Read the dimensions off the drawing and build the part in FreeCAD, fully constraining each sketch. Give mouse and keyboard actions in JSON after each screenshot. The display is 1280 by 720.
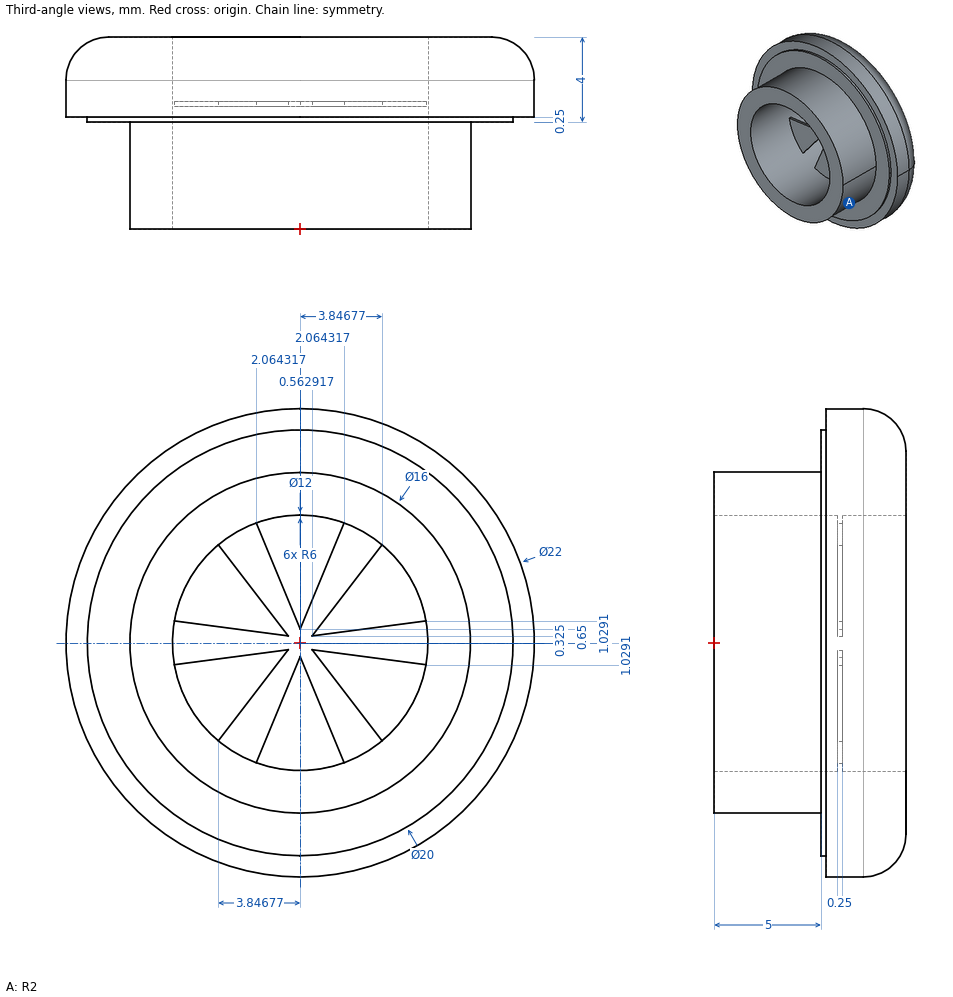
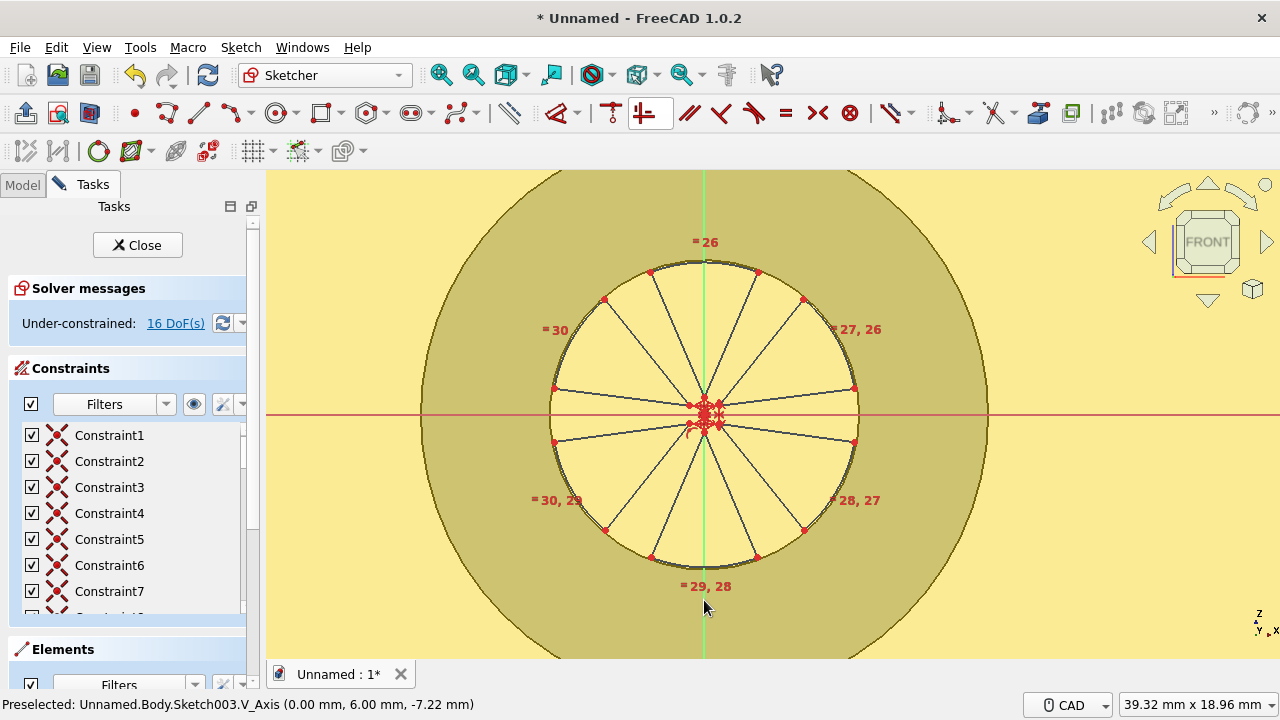
{"action": "left_click", "coordinate": [556, 114]}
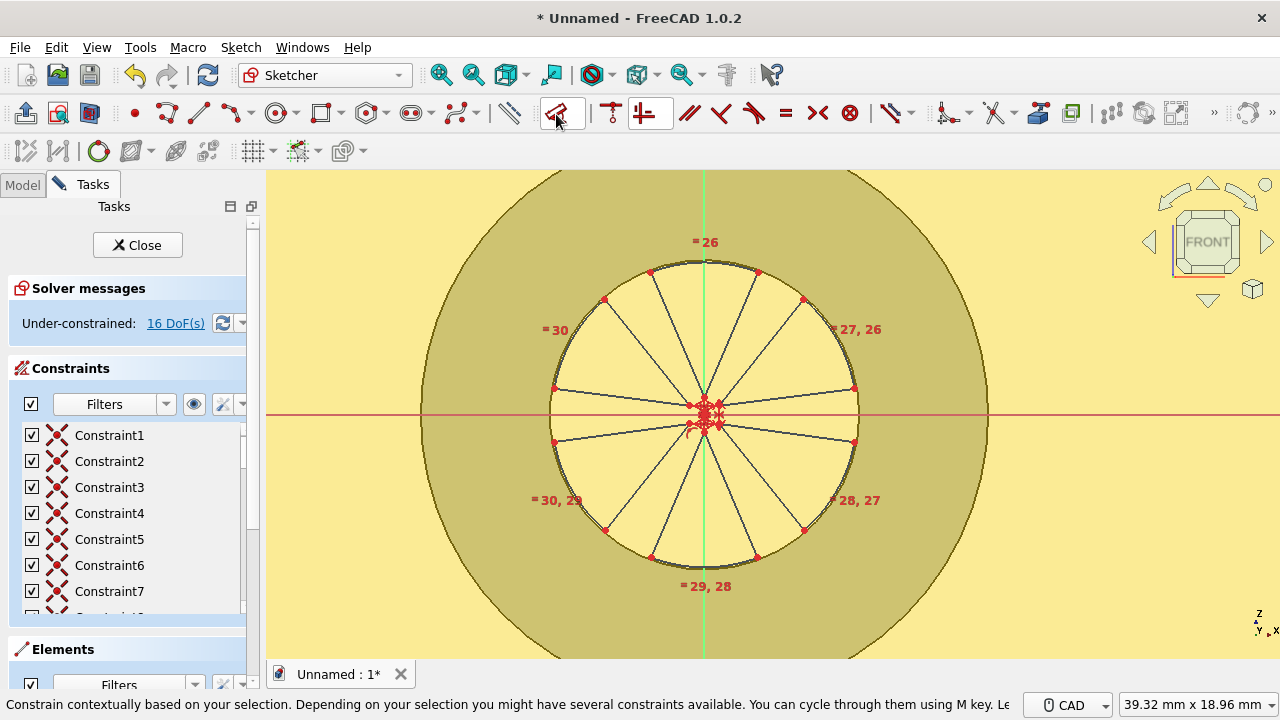
{"action": "left_click", "coordinate": [726, 264]}
{"action": "left_click", "coordinate": [731, 232]}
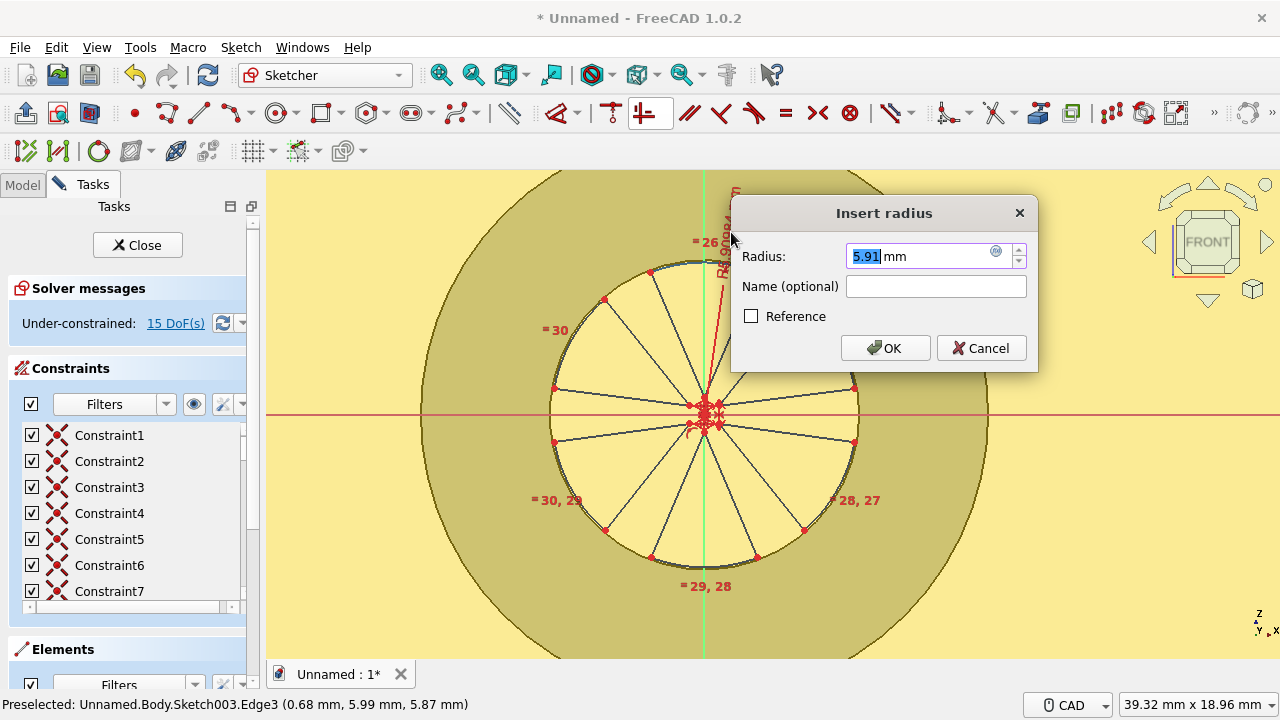
{"action": "type", "text": "6"}
{"action": "key", "text": "Return"}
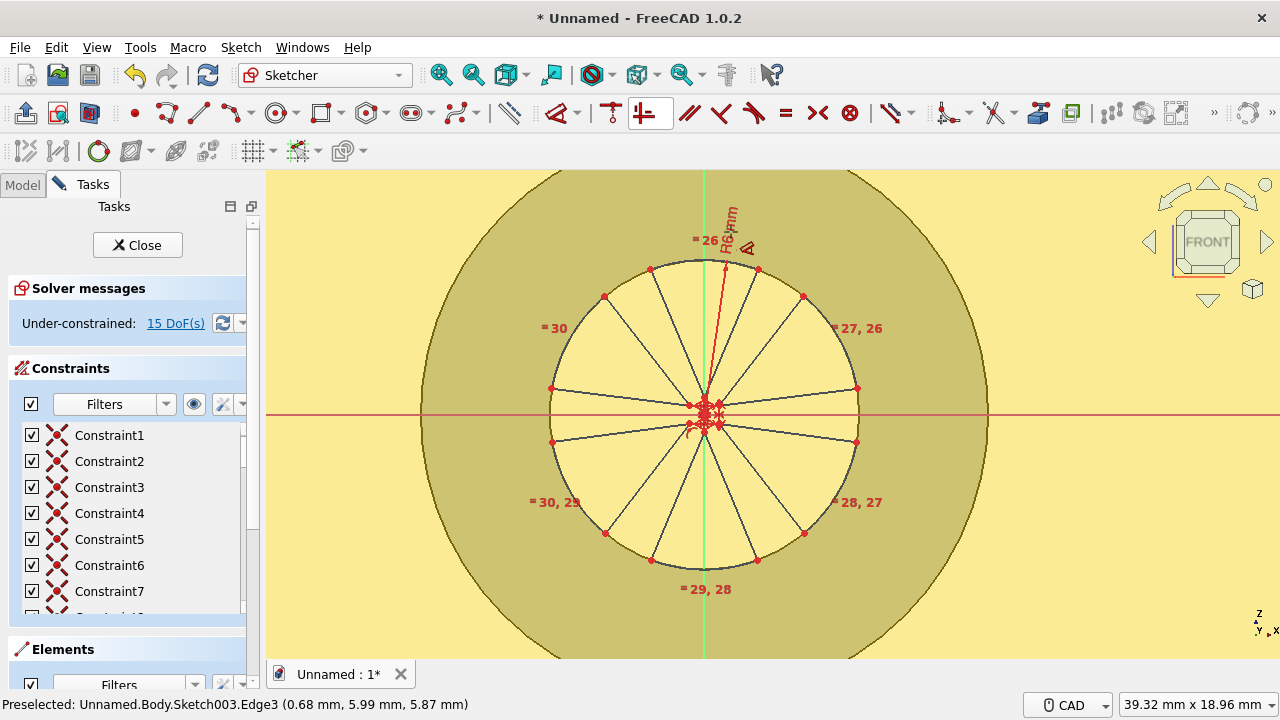
{"action": "scroll", "coordinate": [704, 397], "scroll_direction": "up", "scroll_amount": 5}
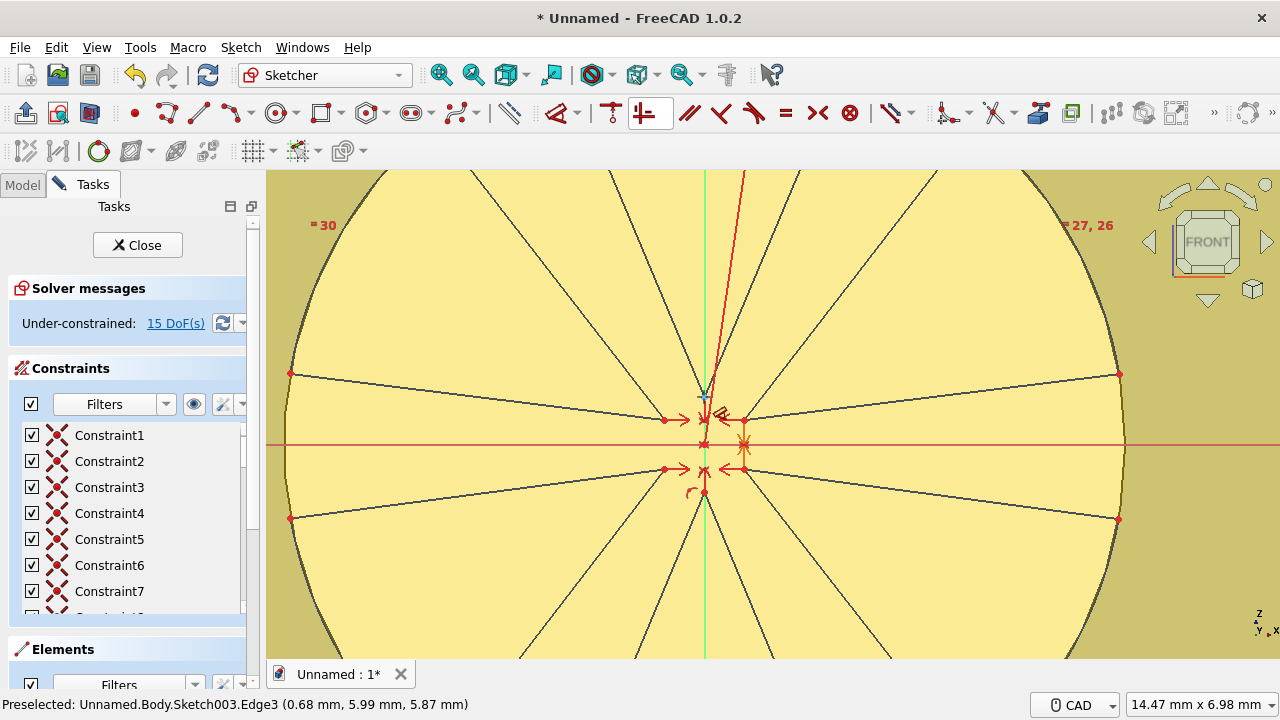
{"action": "left_click", "coordinate": [705, 397]}
{"action": "left_click", "coordinate": [739, 404]}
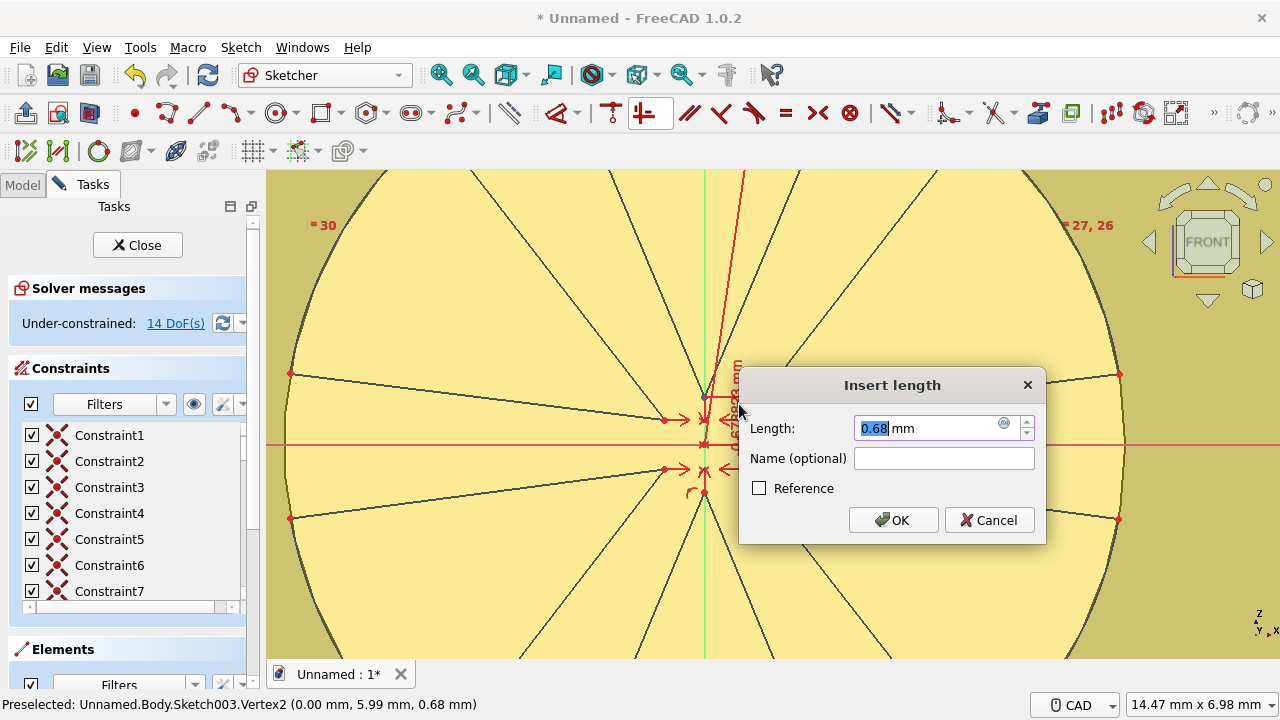
{"action": "type", "text": "0.65"}
{"action": "key", "text": "Return"}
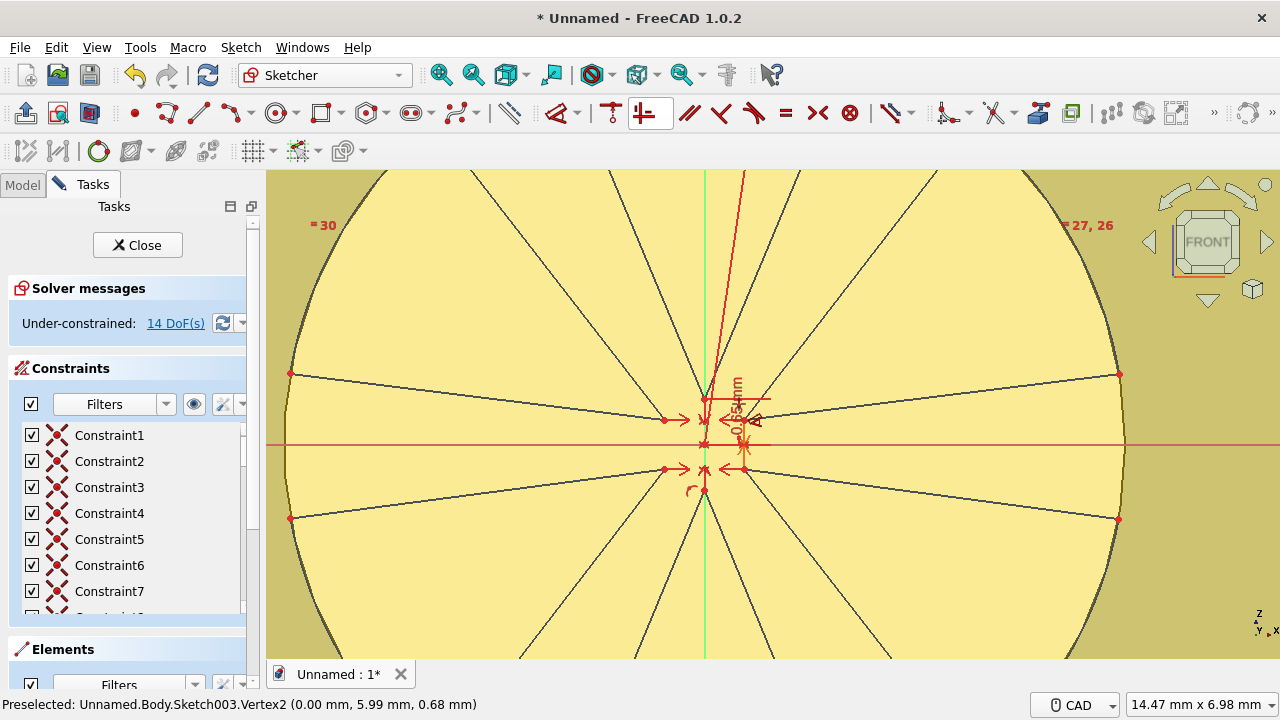
{"action": "scroll", "coordinate": [744, 420], "scroll_direction": "up", "scroll_amount": 3}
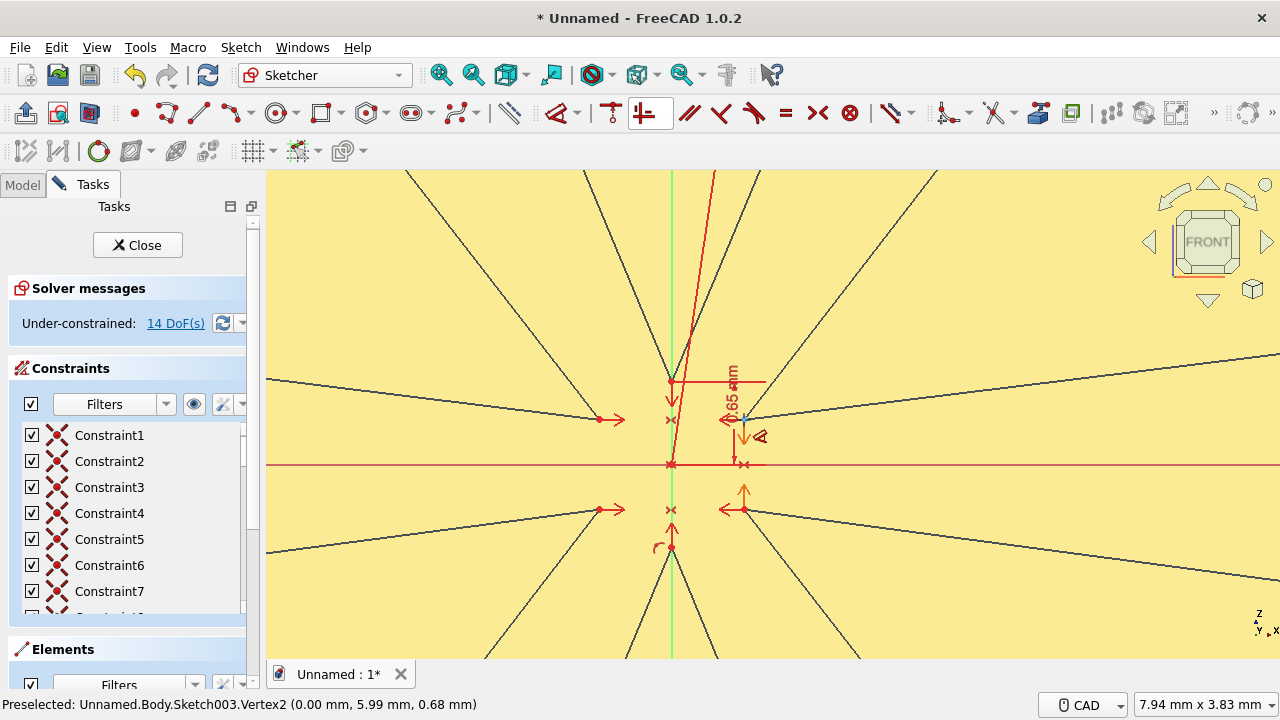
{"action": "left_click", "coordinate": [744, 420]}
{"action": "left_click", "coordinate": [778, 442]}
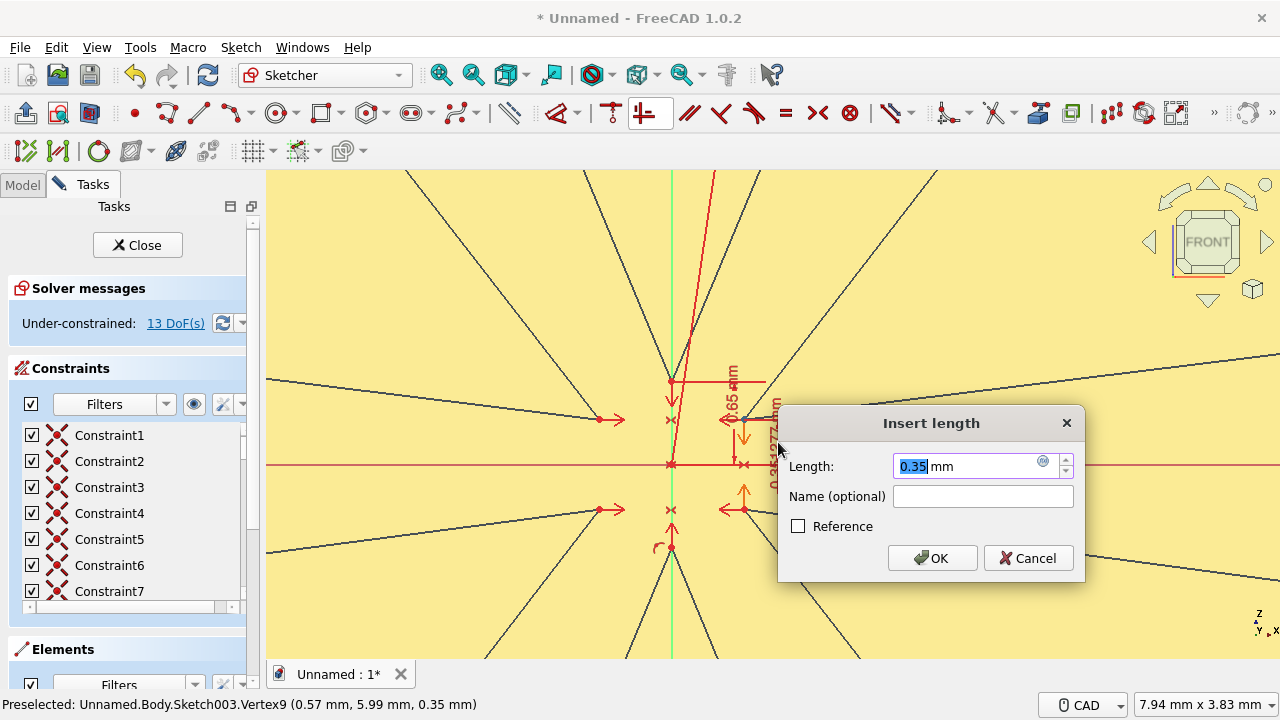
{"action": "type", "text": "0.325"}
{"action": "key", "text": "Return"}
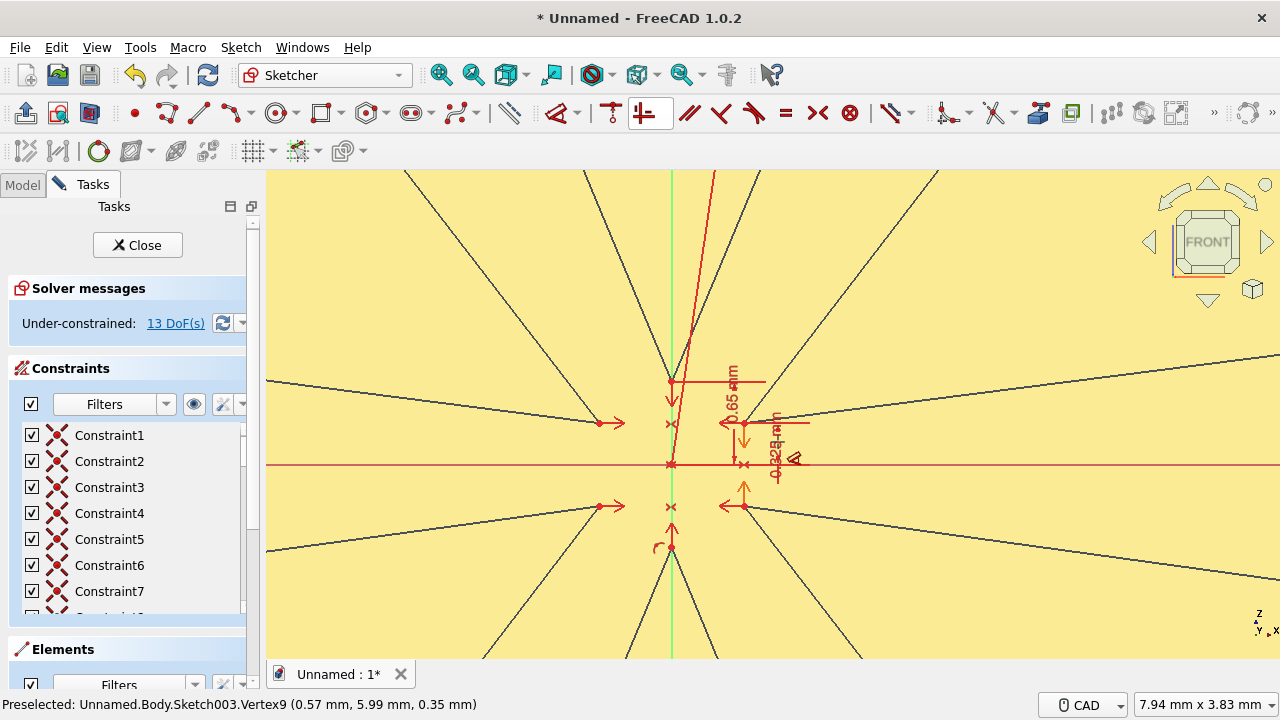
{"action": "scroll", "coordinate": [713, 402], "scroll_direction": "down", "scroll_amount": 8}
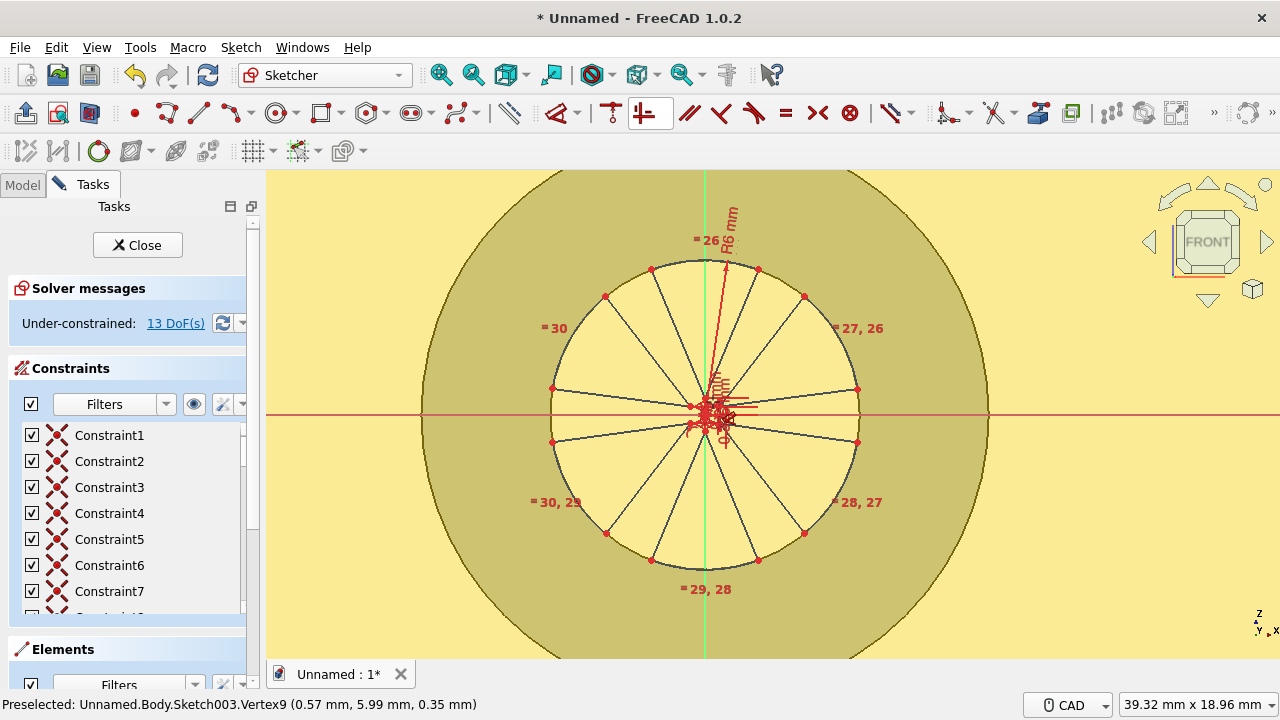
{"action": "scroll", "coordinate": [858, 389], "scroll_direction": "up", "scroll_amount": 3}